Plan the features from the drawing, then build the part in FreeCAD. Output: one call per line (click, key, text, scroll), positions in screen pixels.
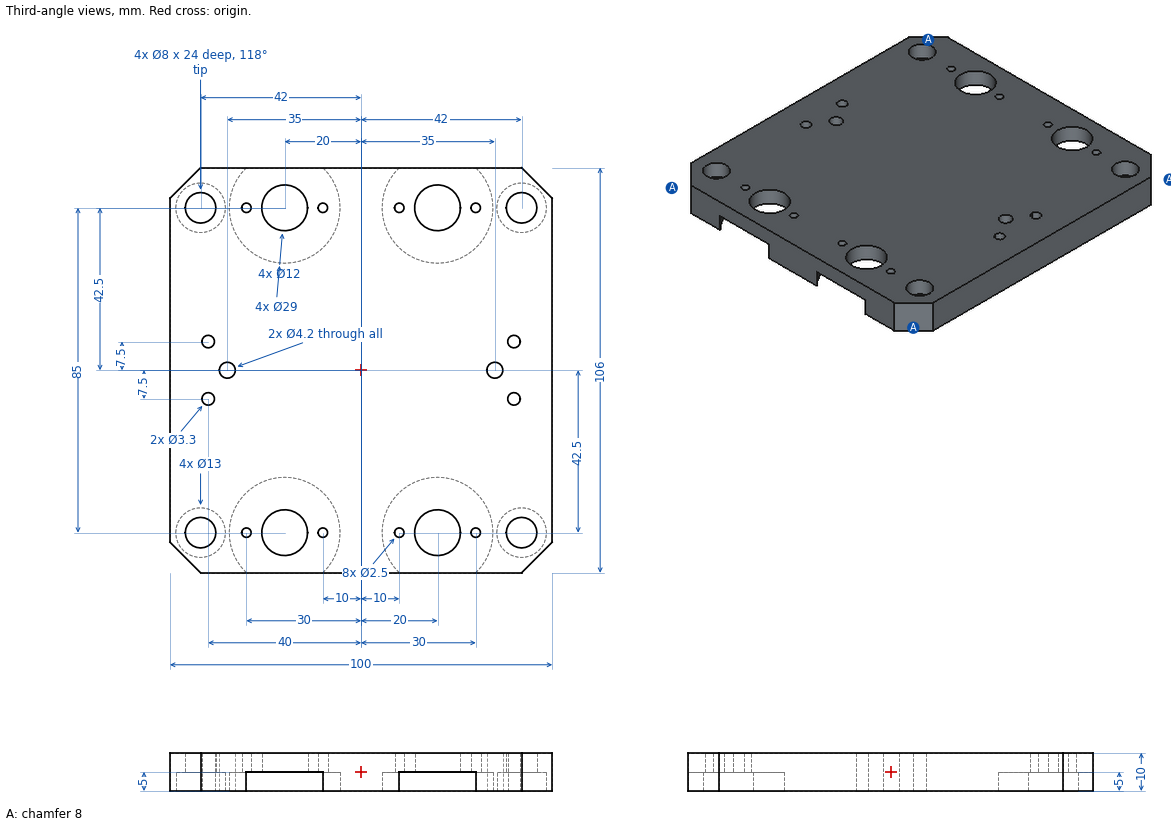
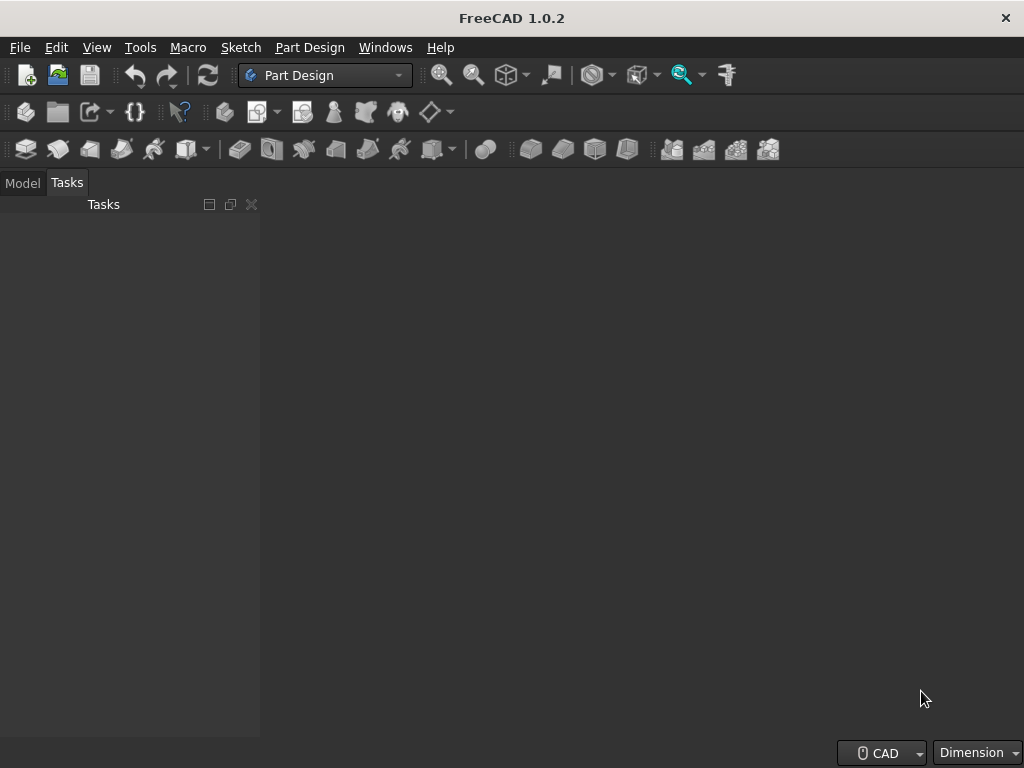
click(26, 76)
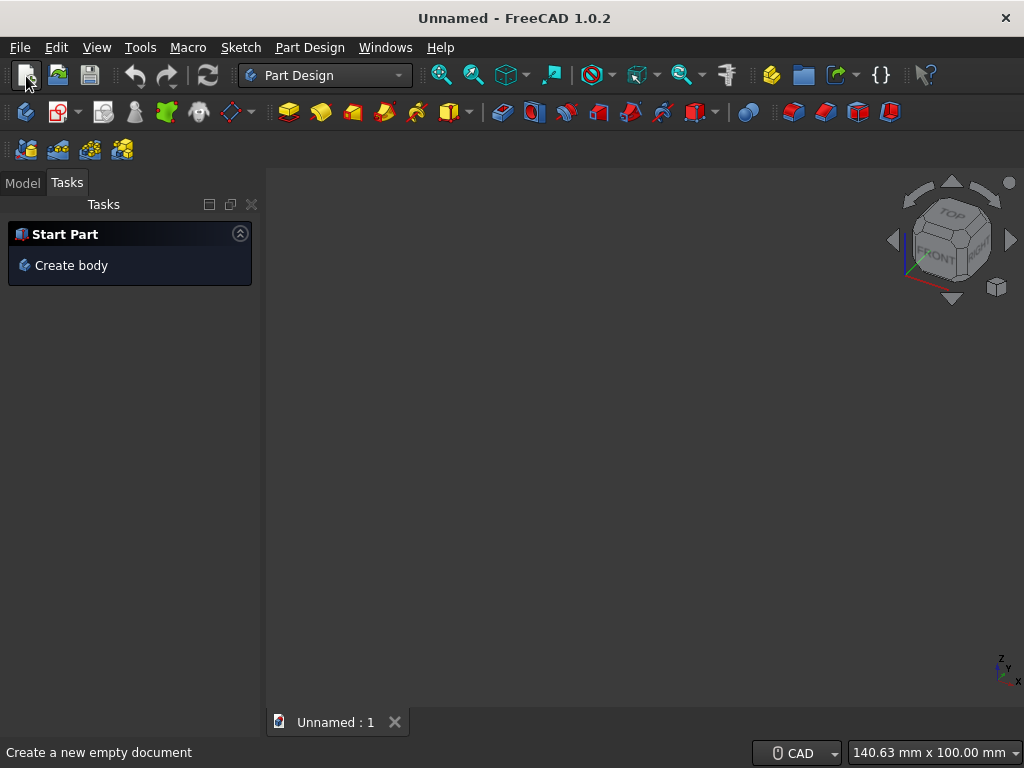
click(58, 112)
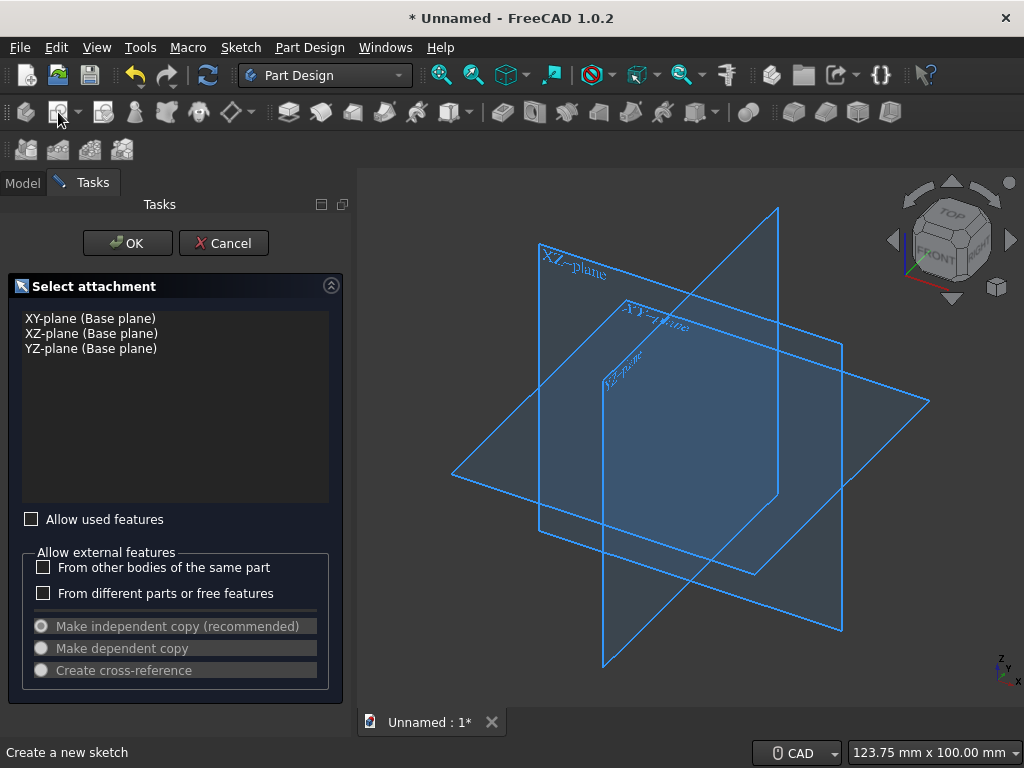
click(82, 318)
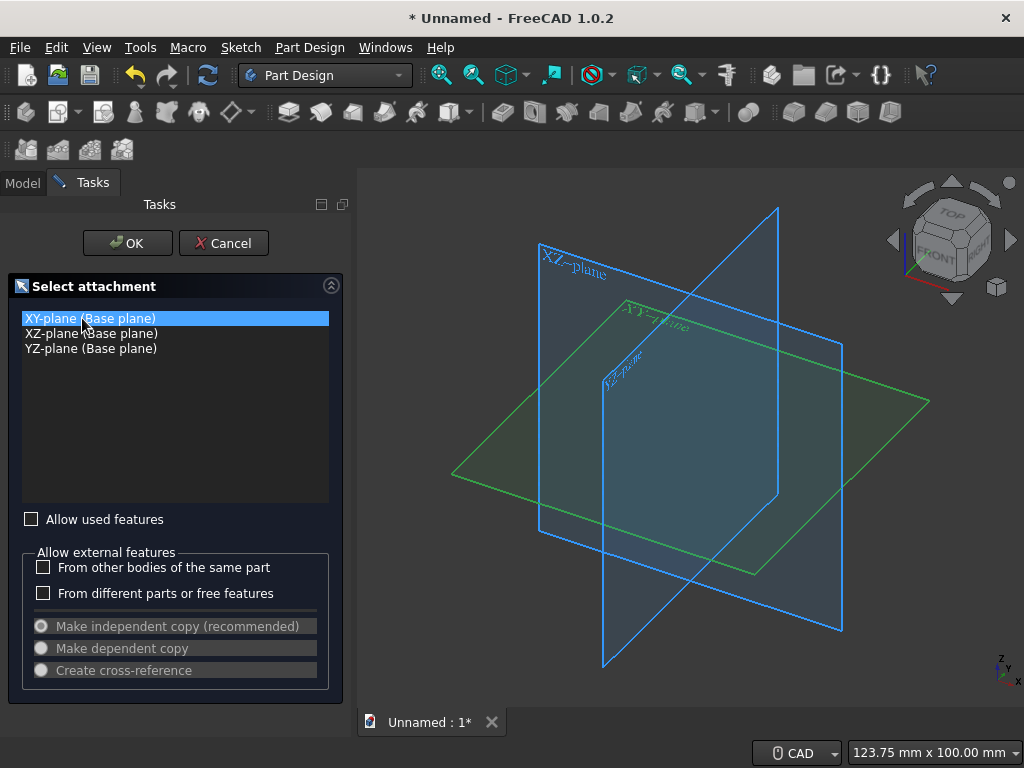
click(128, 243)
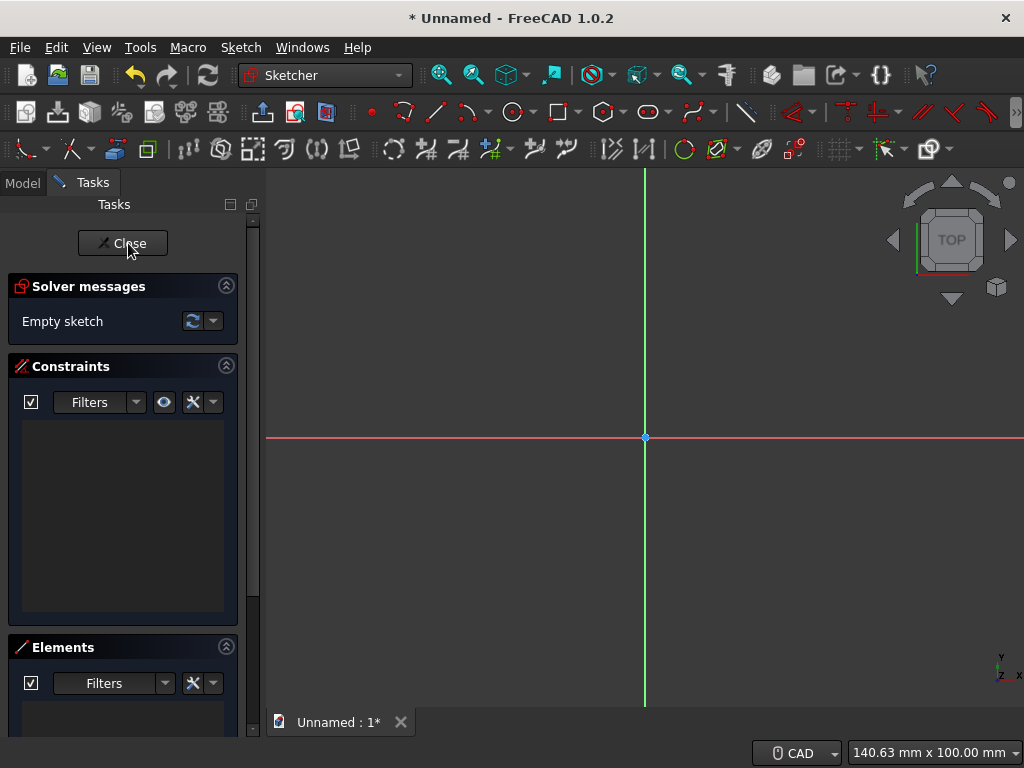
scroll(493, 438, down, 3)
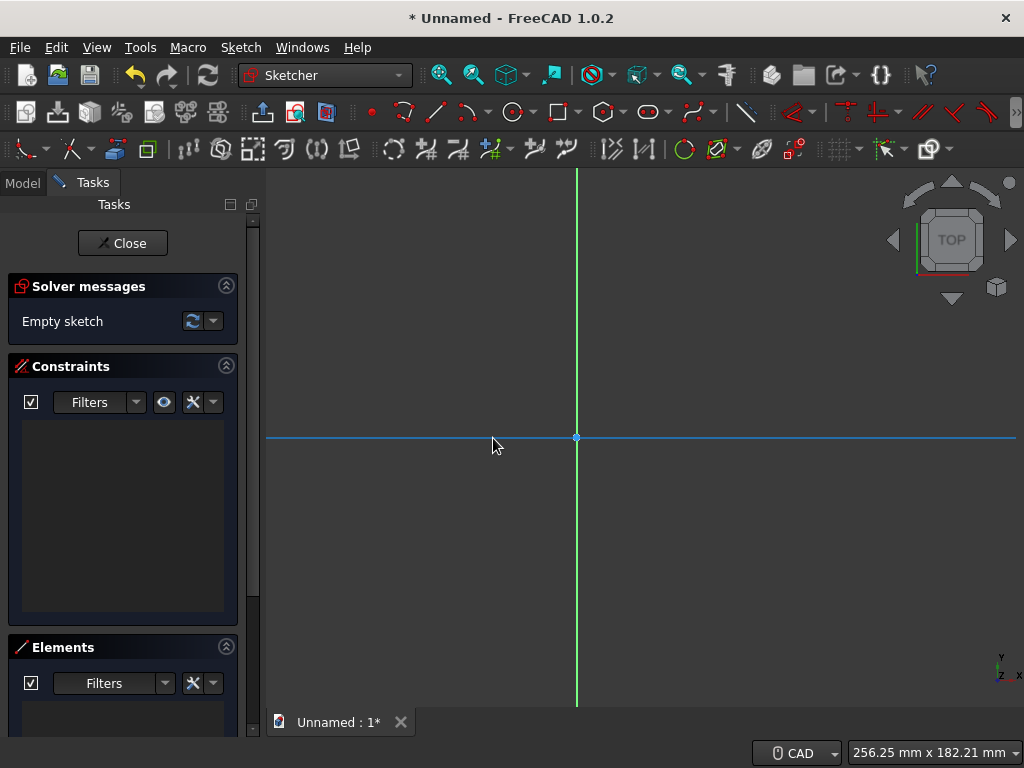
click(580, 112)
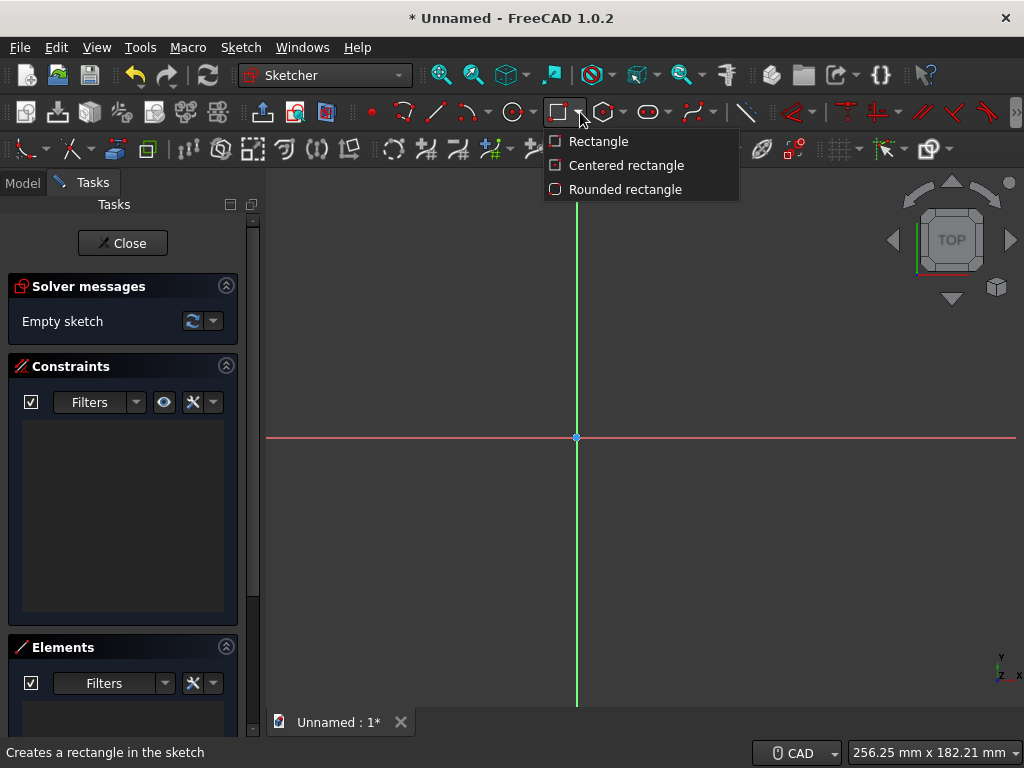
click(642, 165)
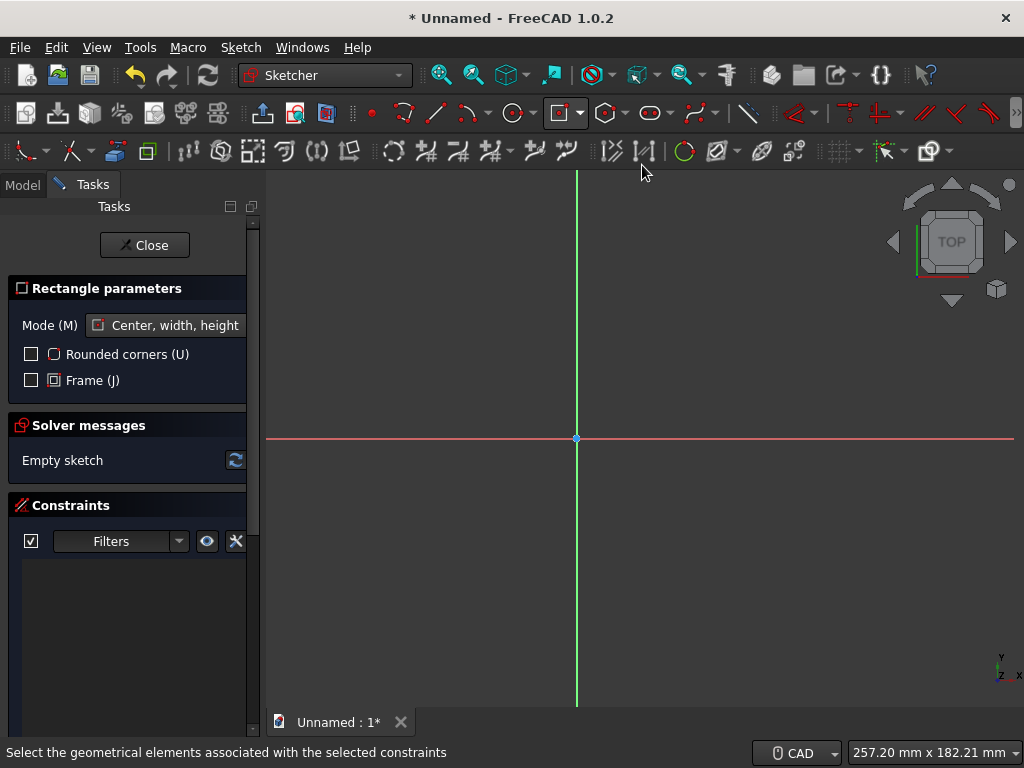
click(577, 439)
move(724, 283)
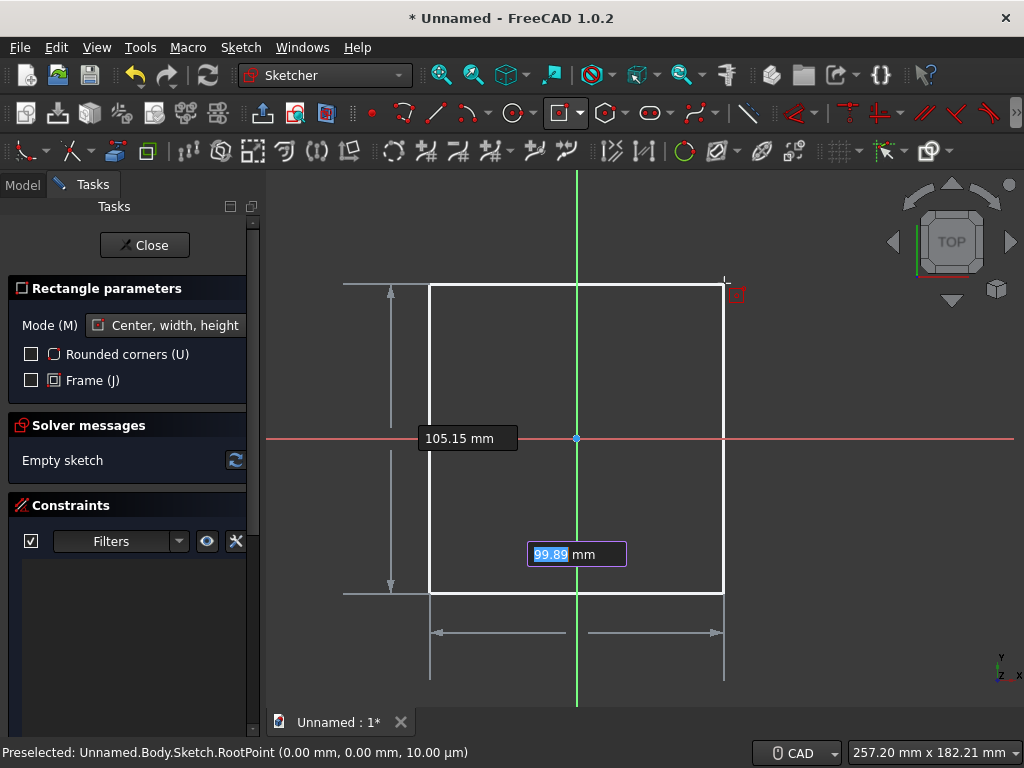
text(100)
key(Tab)
text(106)
key(Return)
key(Escape)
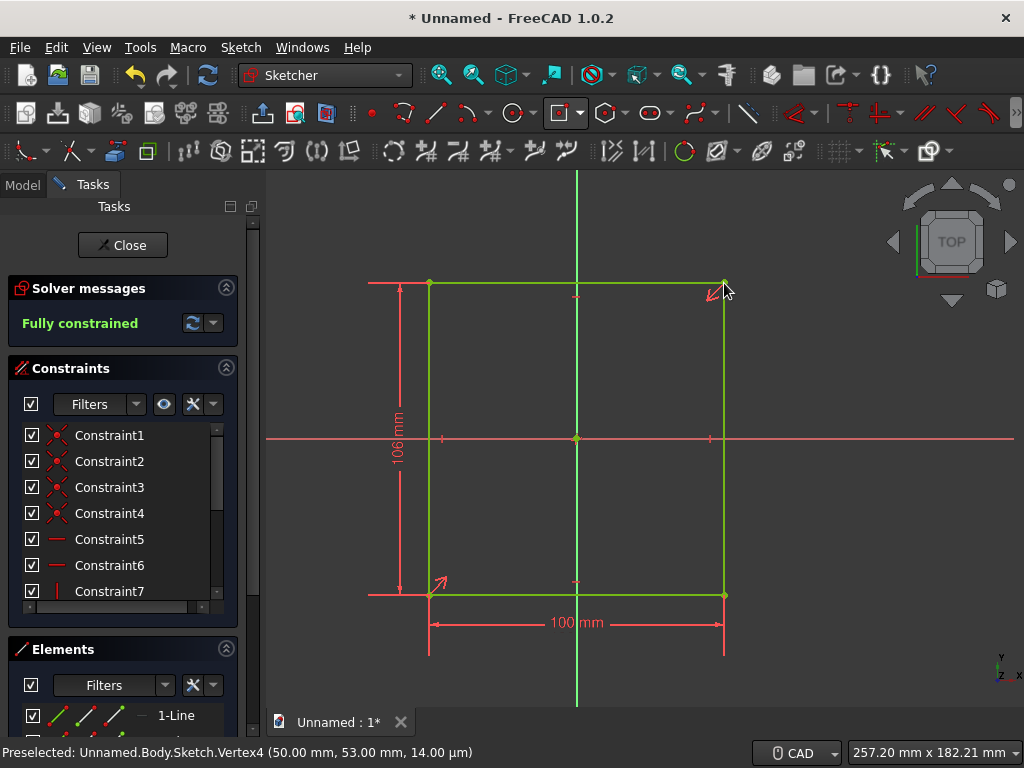
click(123, 245)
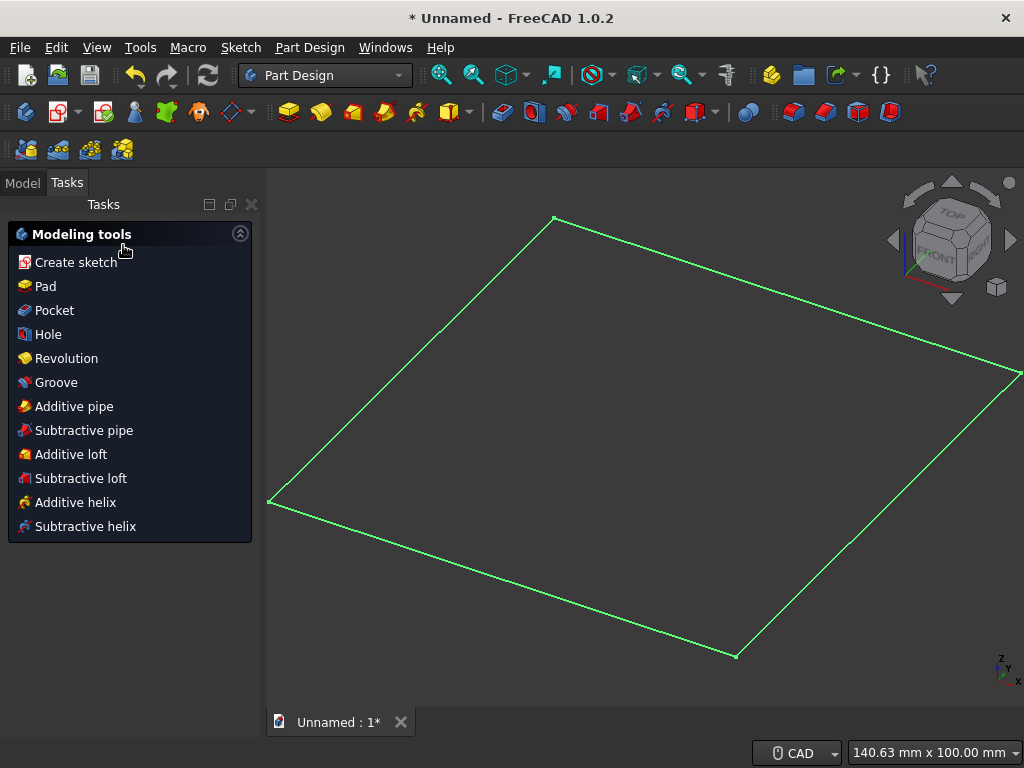
click(290, 112)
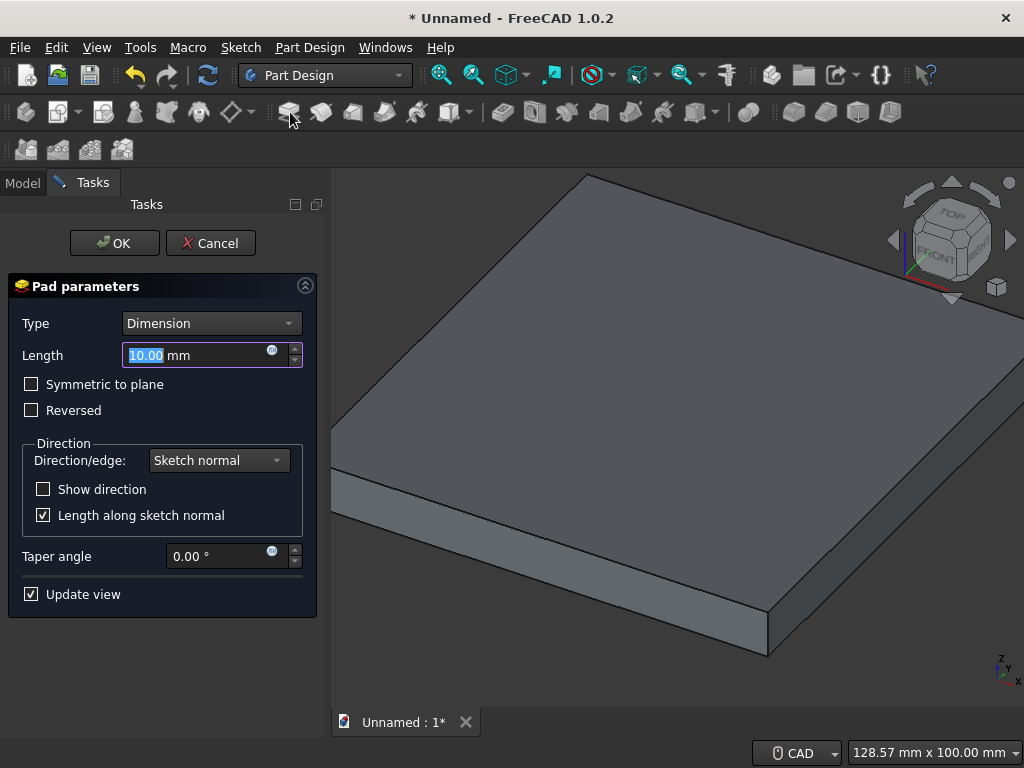
text(10)
key(Tab)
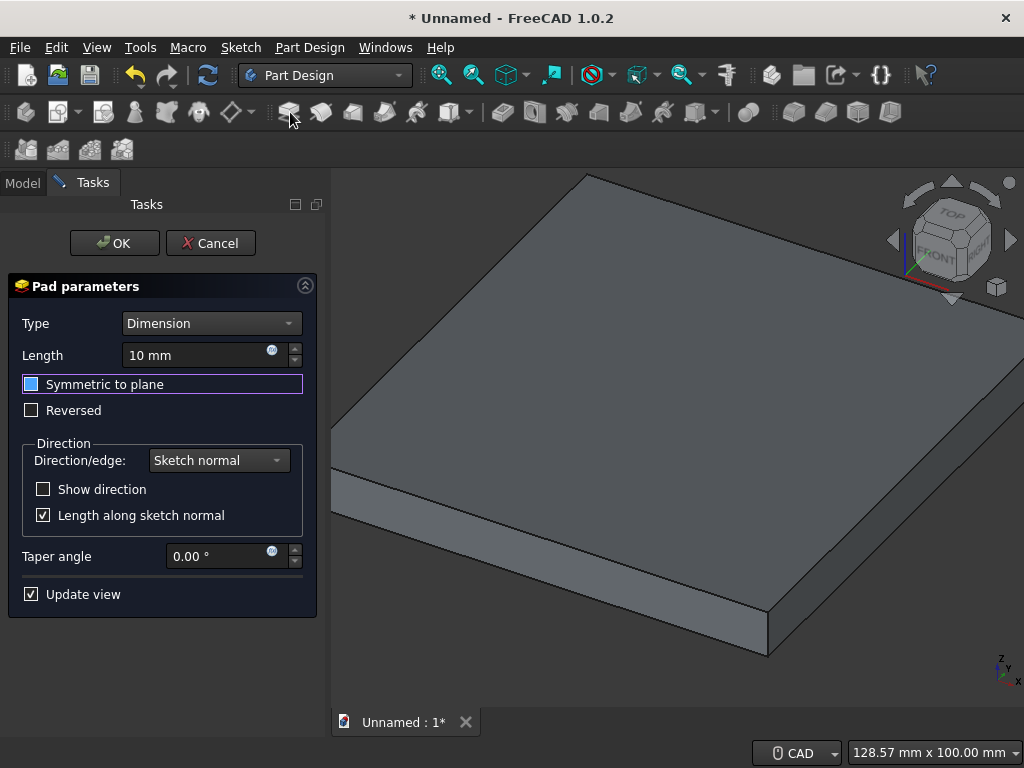
click(30, 384)